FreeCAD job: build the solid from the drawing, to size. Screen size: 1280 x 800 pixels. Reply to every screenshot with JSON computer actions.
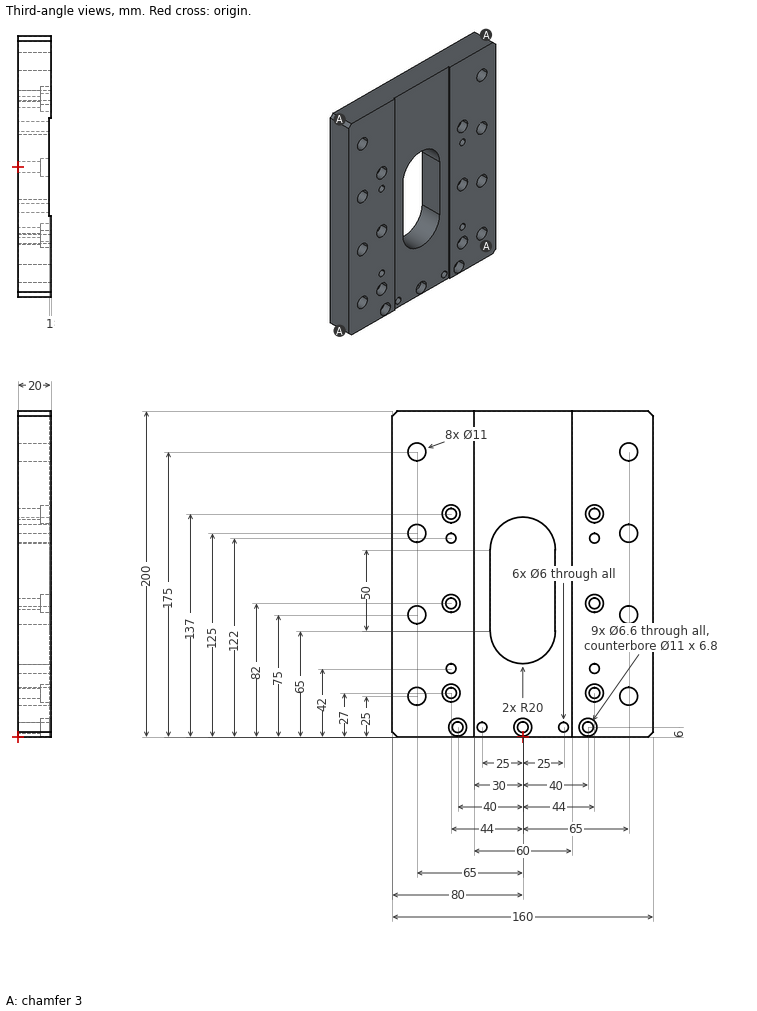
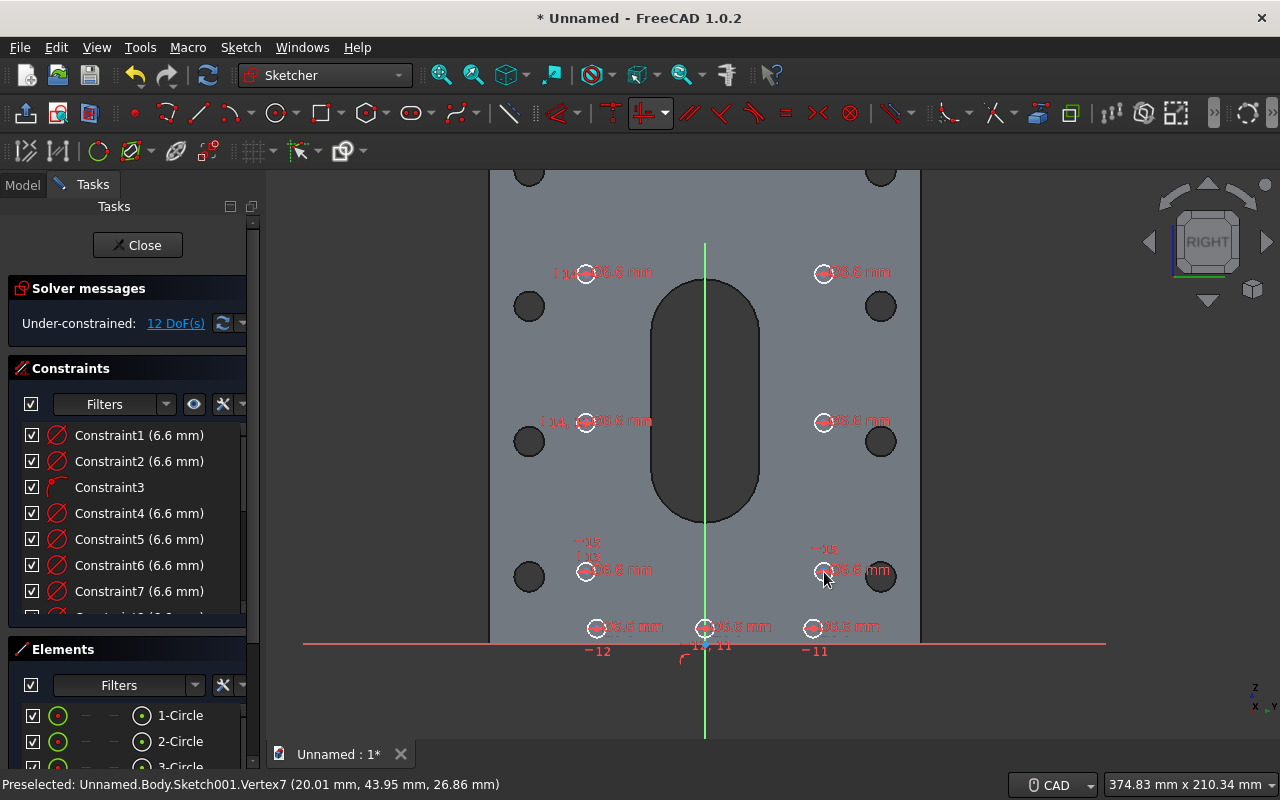
{"action": "left_click", "coordinate": [824, 572]}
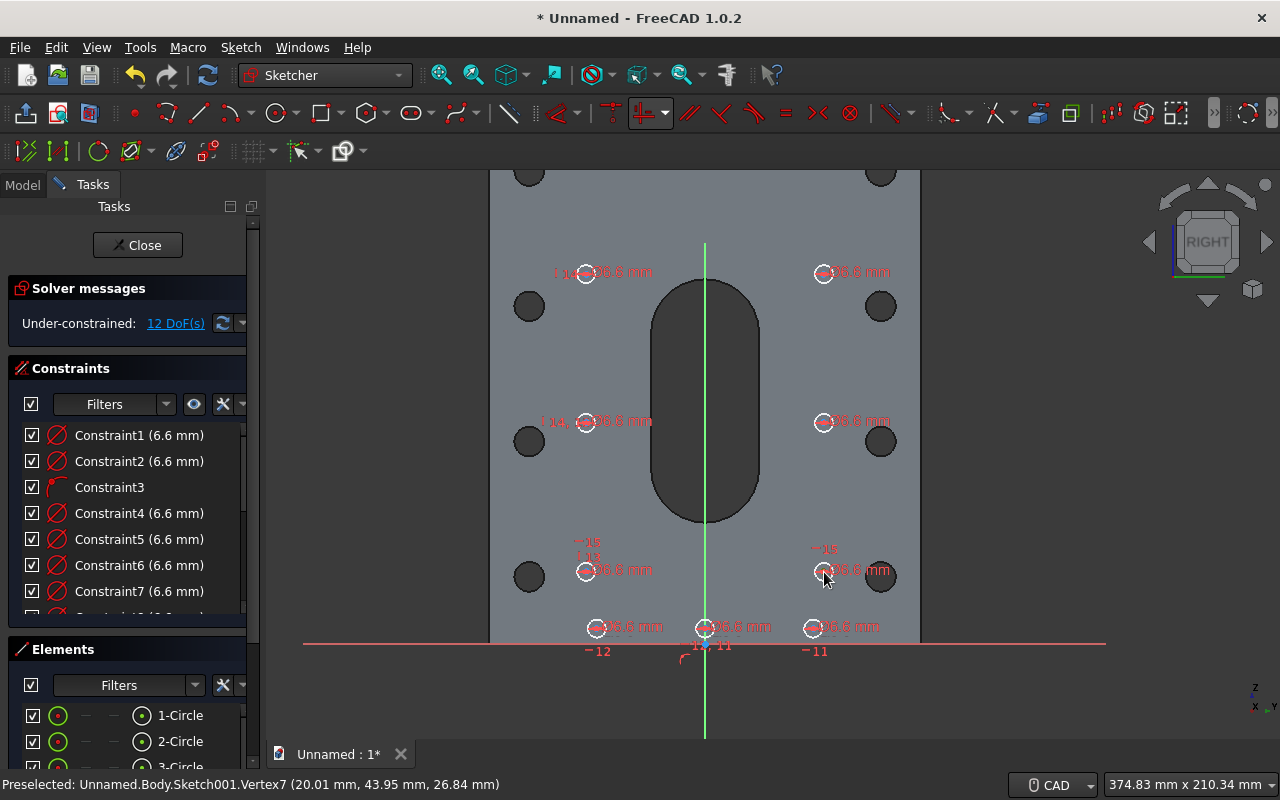
{"action": "left_click", "coordinate": [824, 423]}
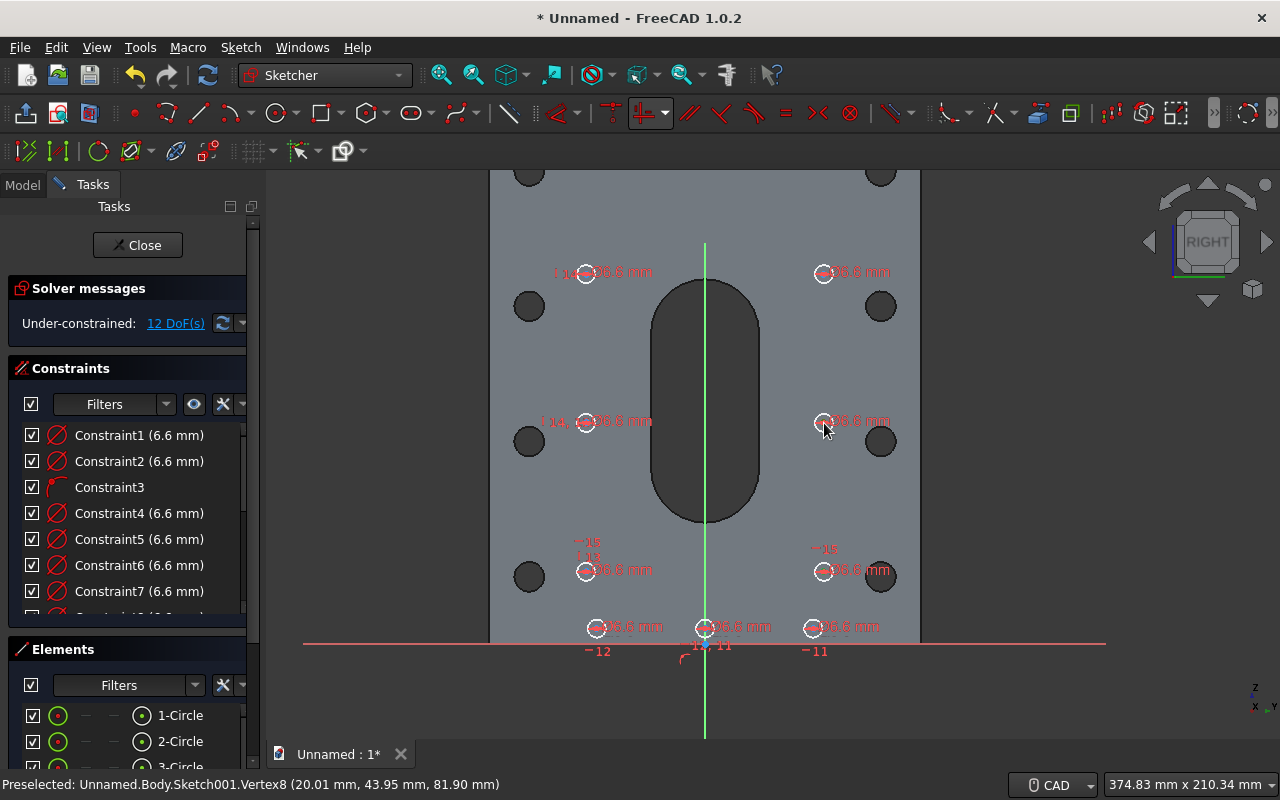
{"action": "key", "text": "v"}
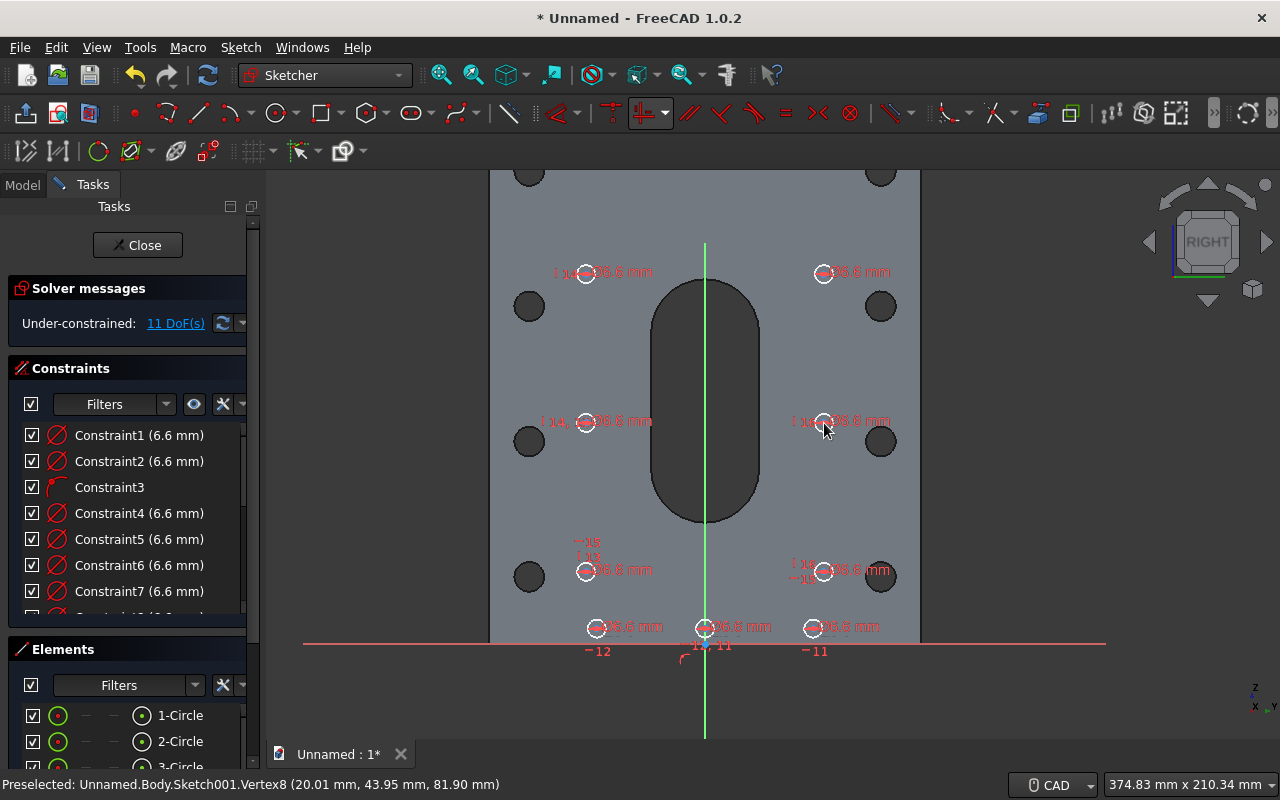
{"action": "left_click", "coordinate": [586, 423]}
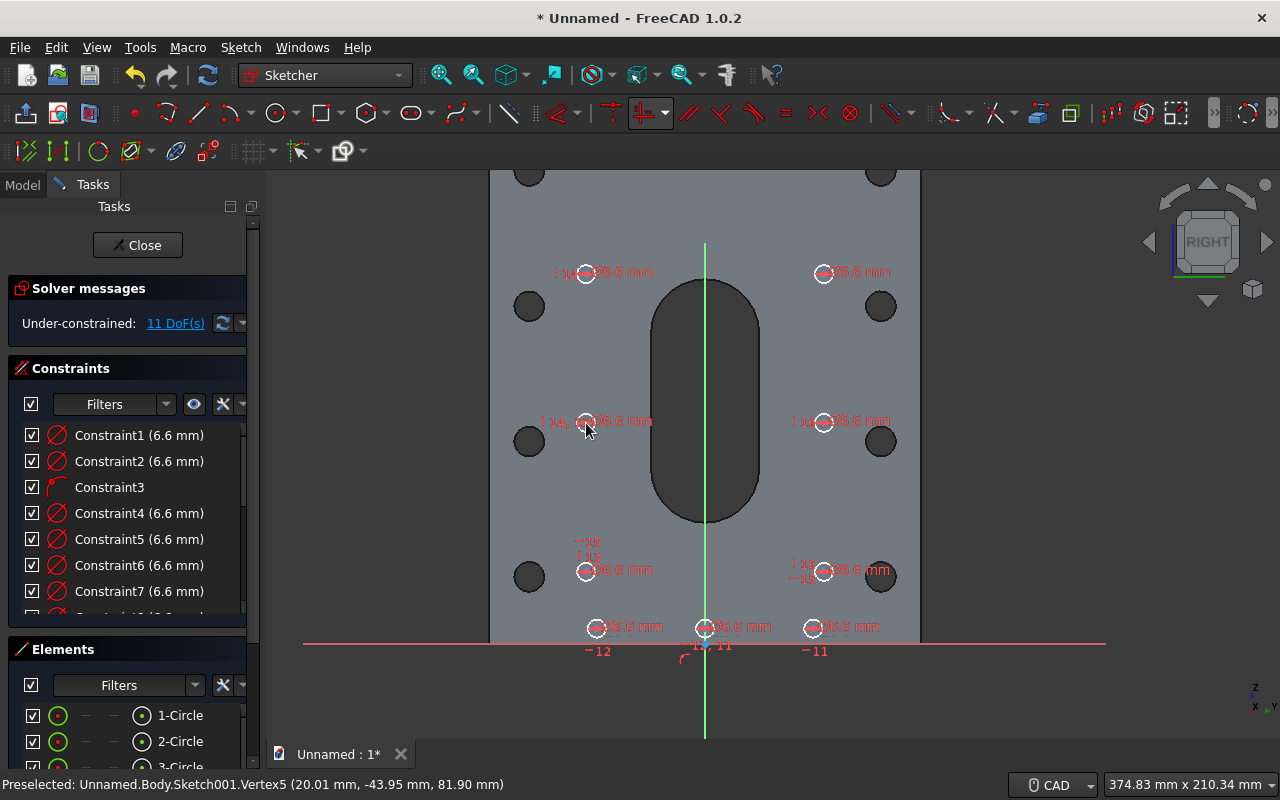
{"action": "left_click", "coordinate": [824, 423]}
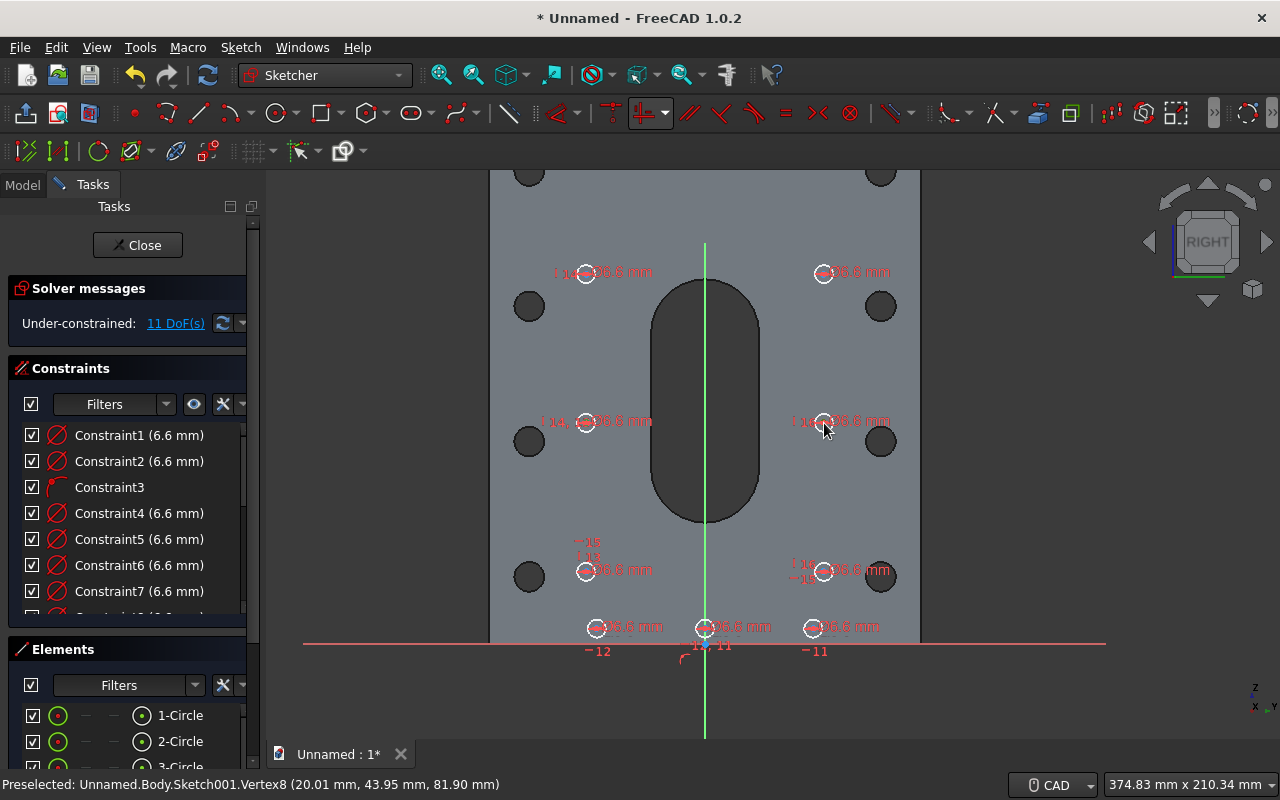
{"action": "left_click", "coordinate": [668, 114]}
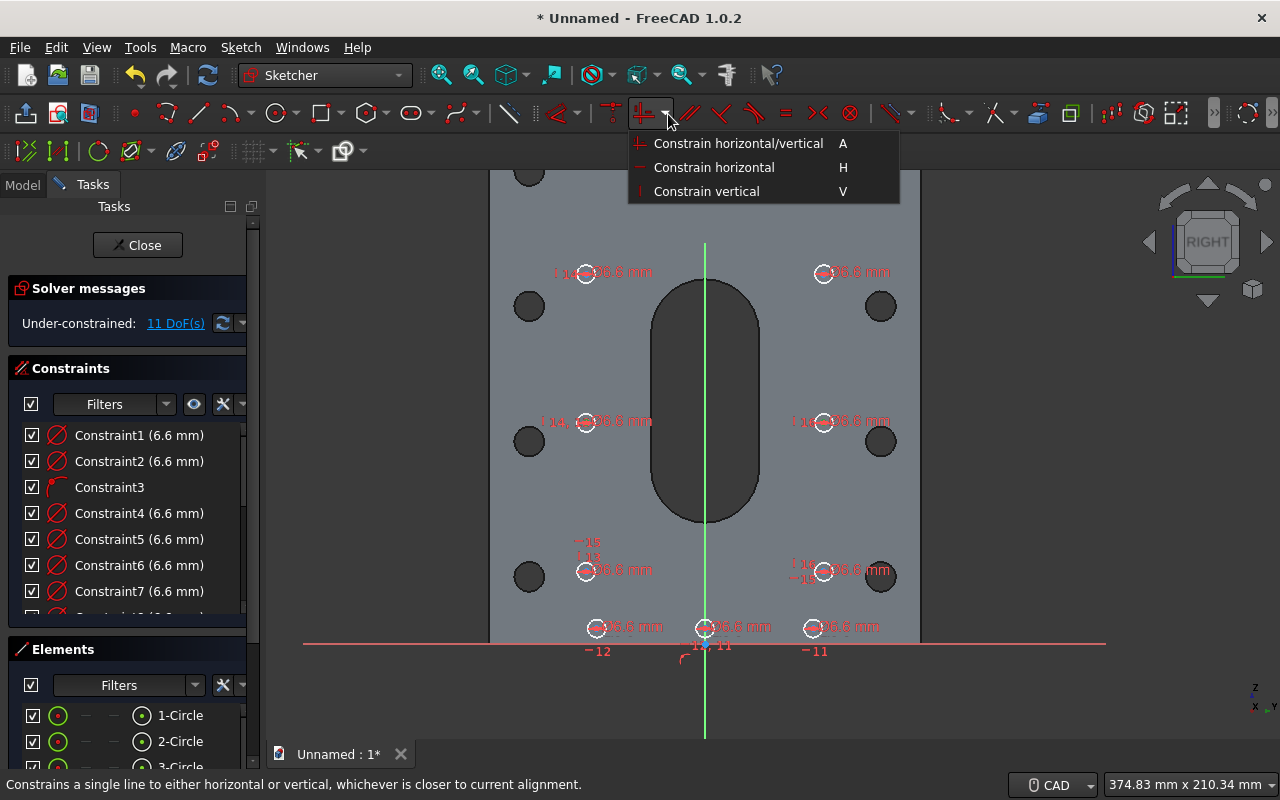
{"action": "left_click", "coordinate": [764, 167]}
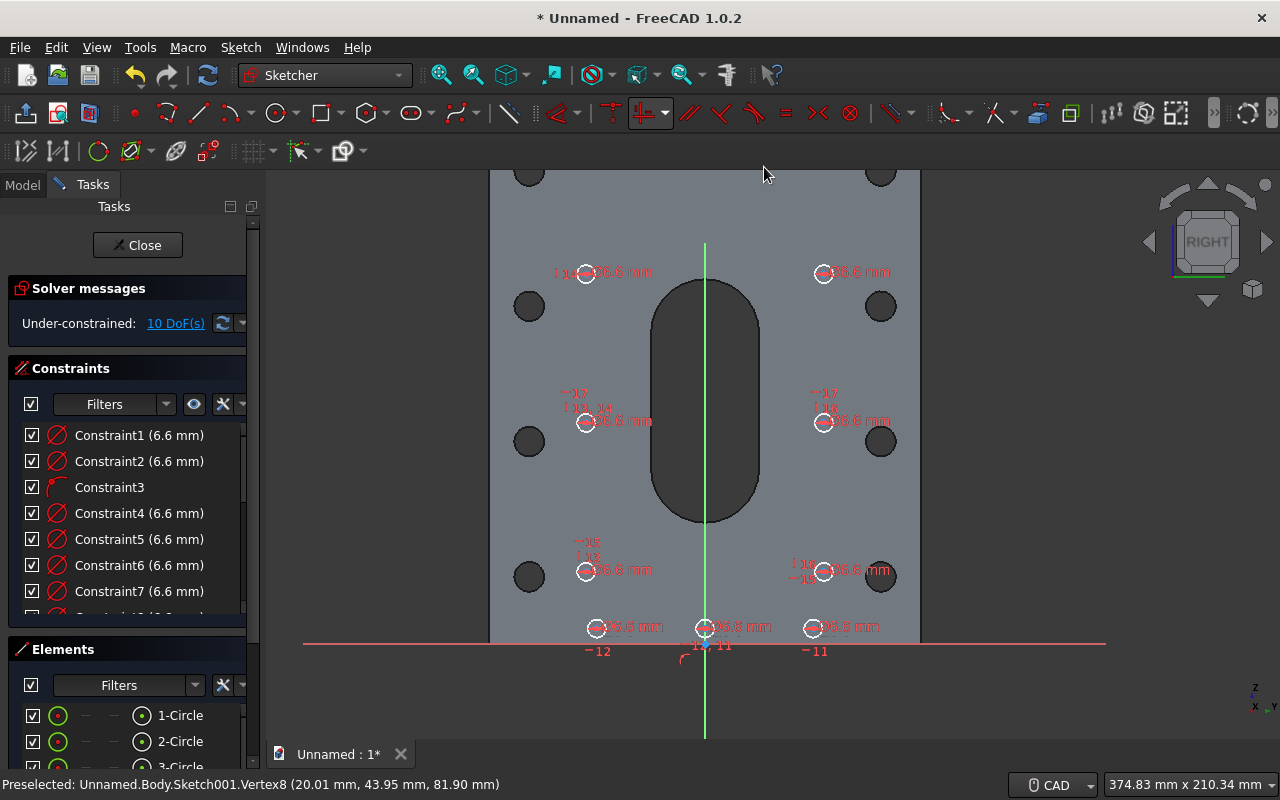
{"action": "left_click", "coordinate": [824, 423]}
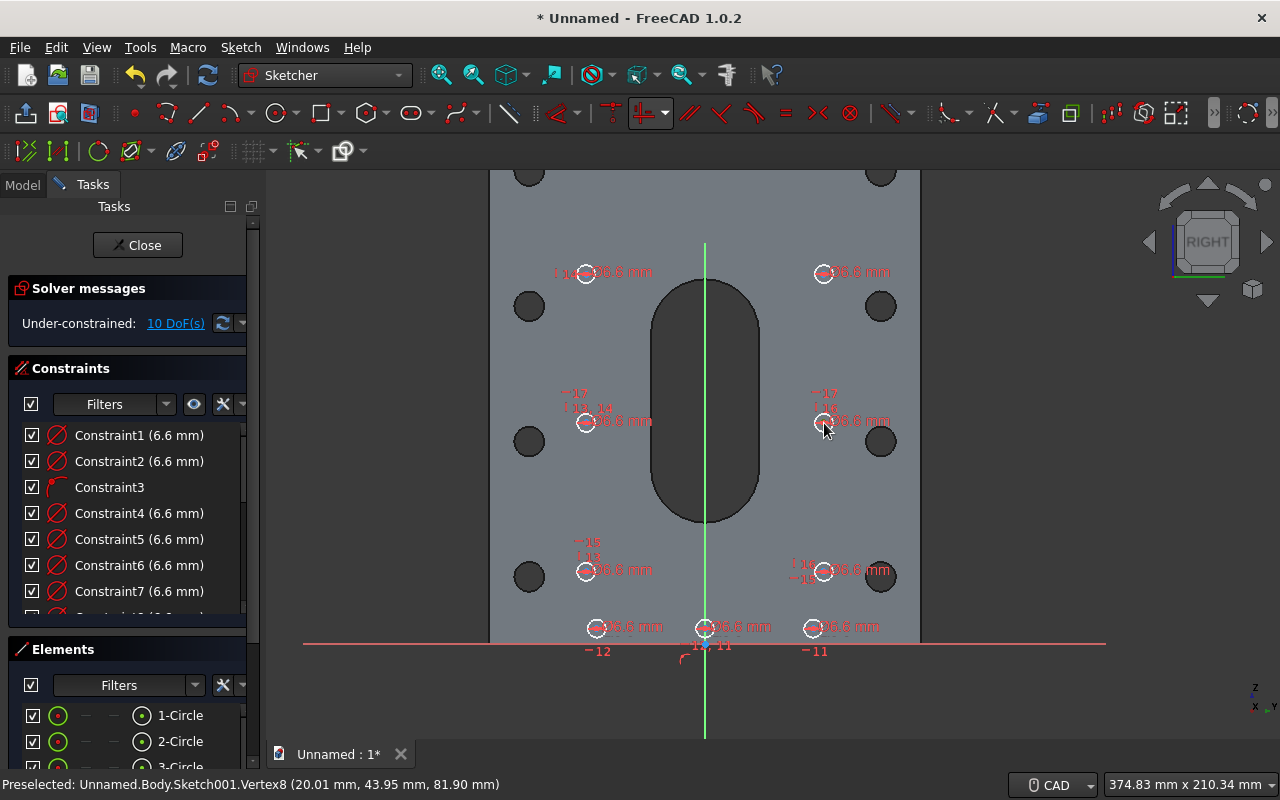
{"action": "left_click", "coordinate": [824, 274]}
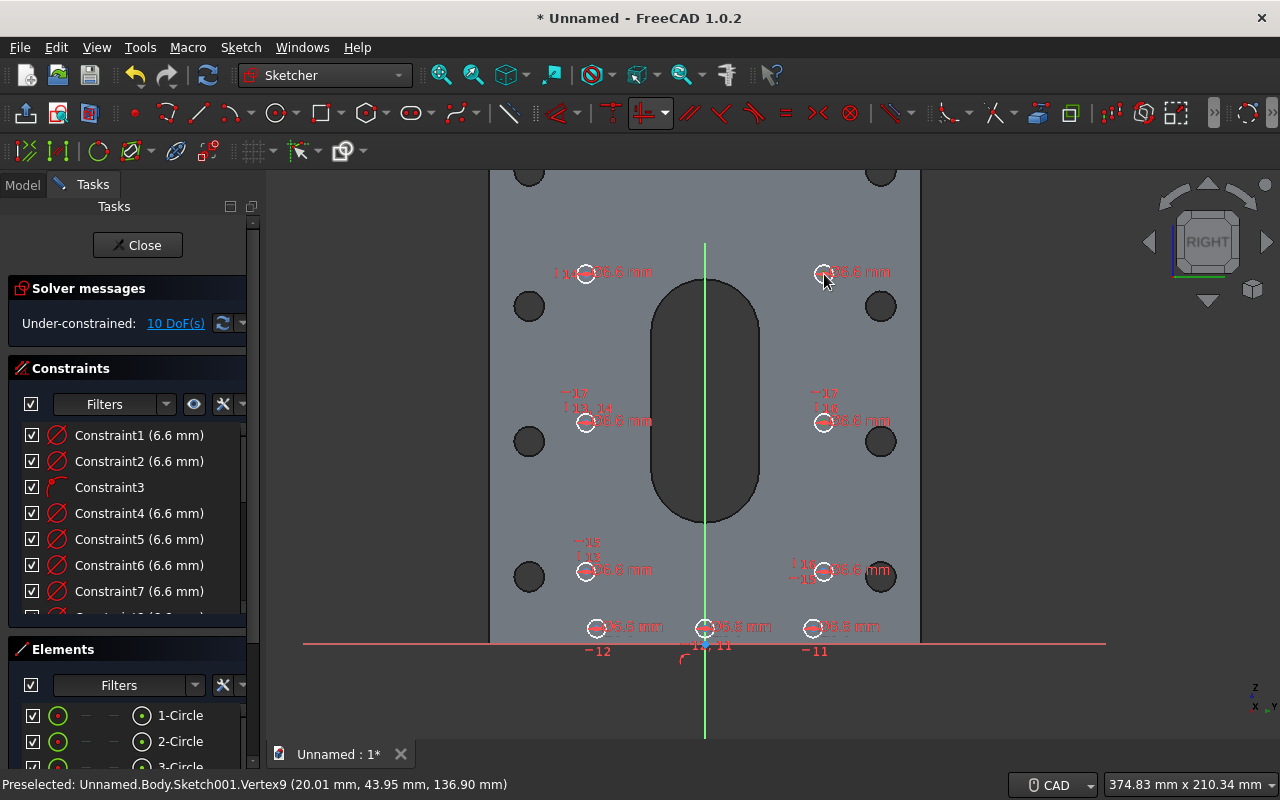
{"action": "key", "text": "v"}